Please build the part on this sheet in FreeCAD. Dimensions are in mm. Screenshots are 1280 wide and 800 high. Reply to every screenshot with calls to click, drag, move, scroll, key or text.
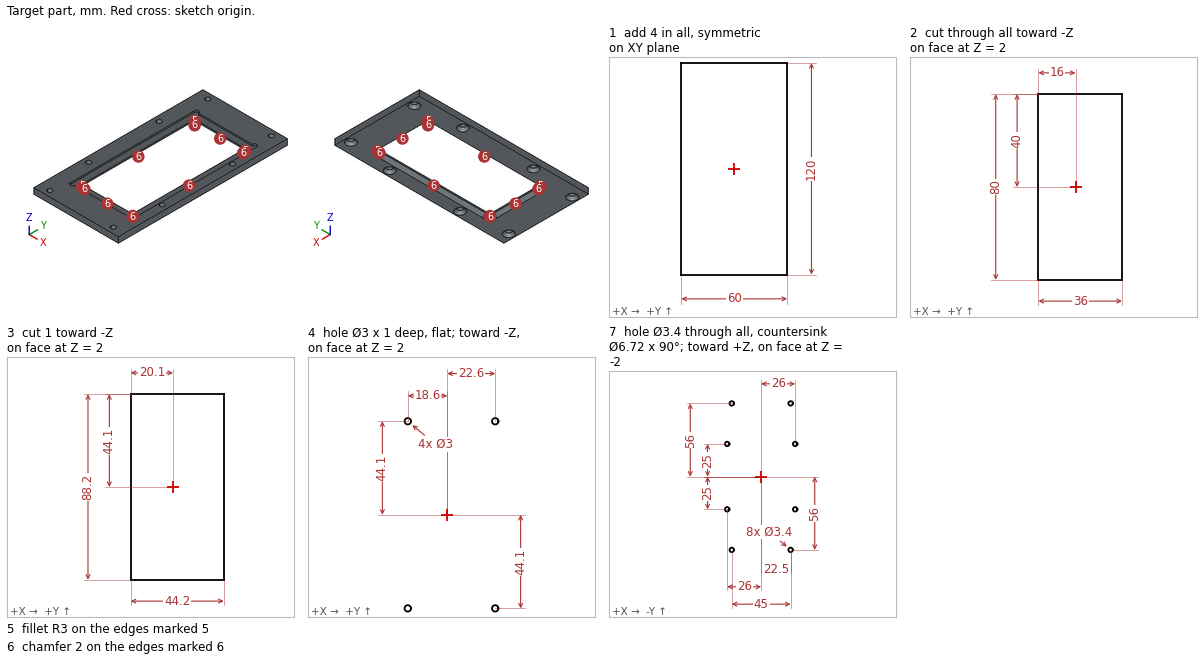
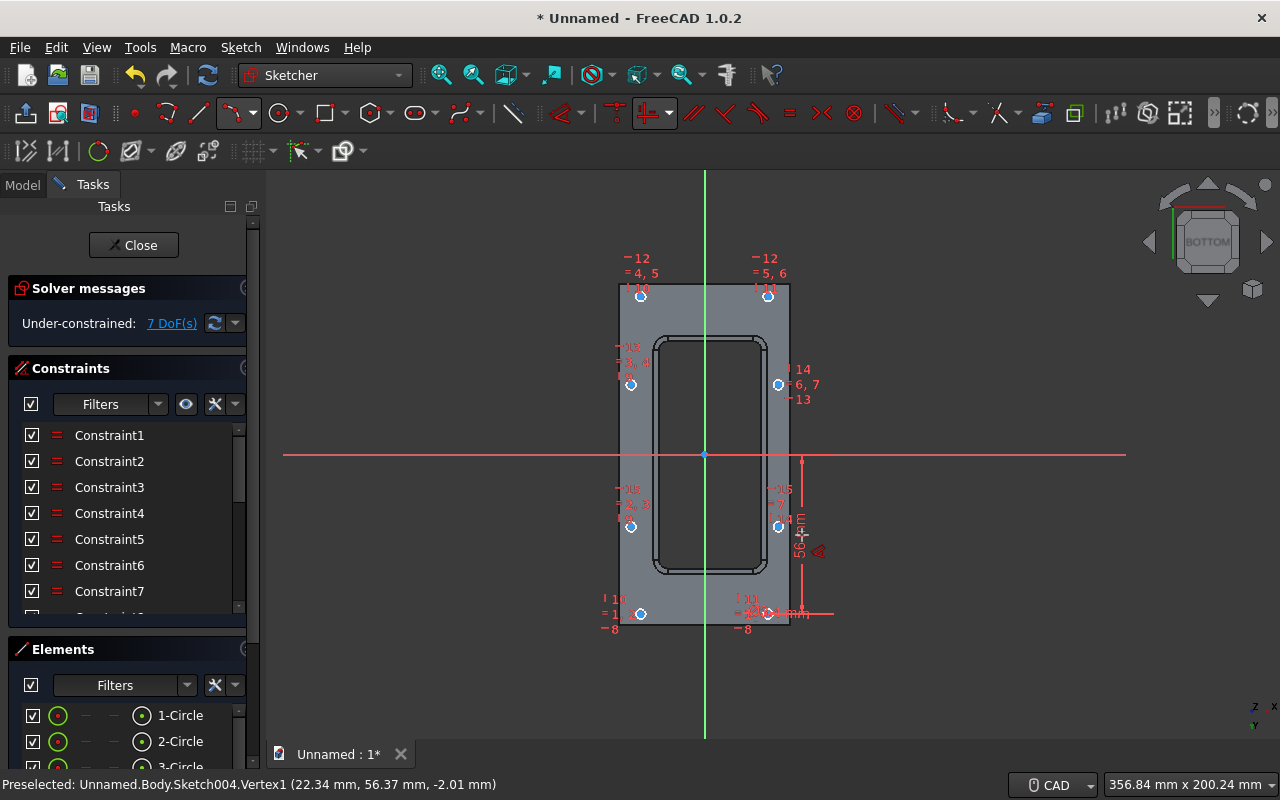
click(631, 527)
click(668, 561)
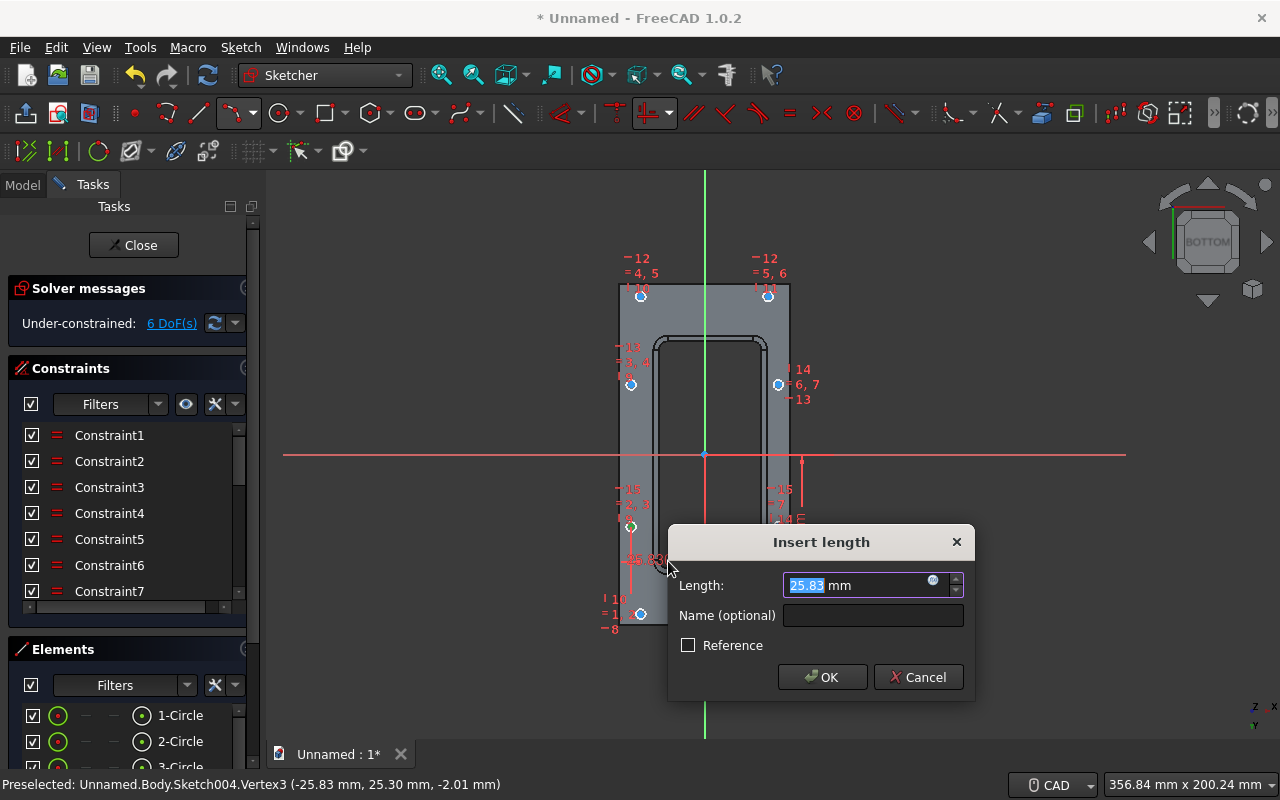
text(26)
key(Return)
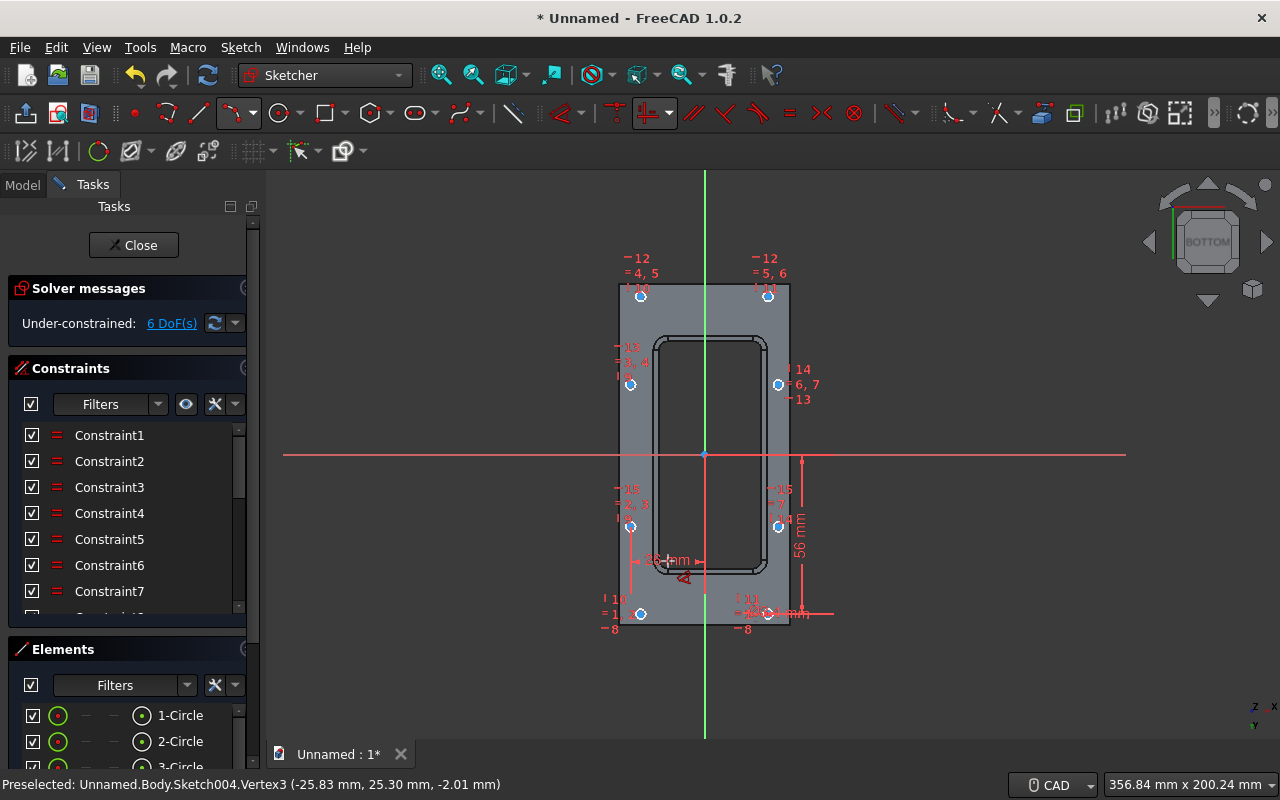
click(631, 527)
click(597, 491)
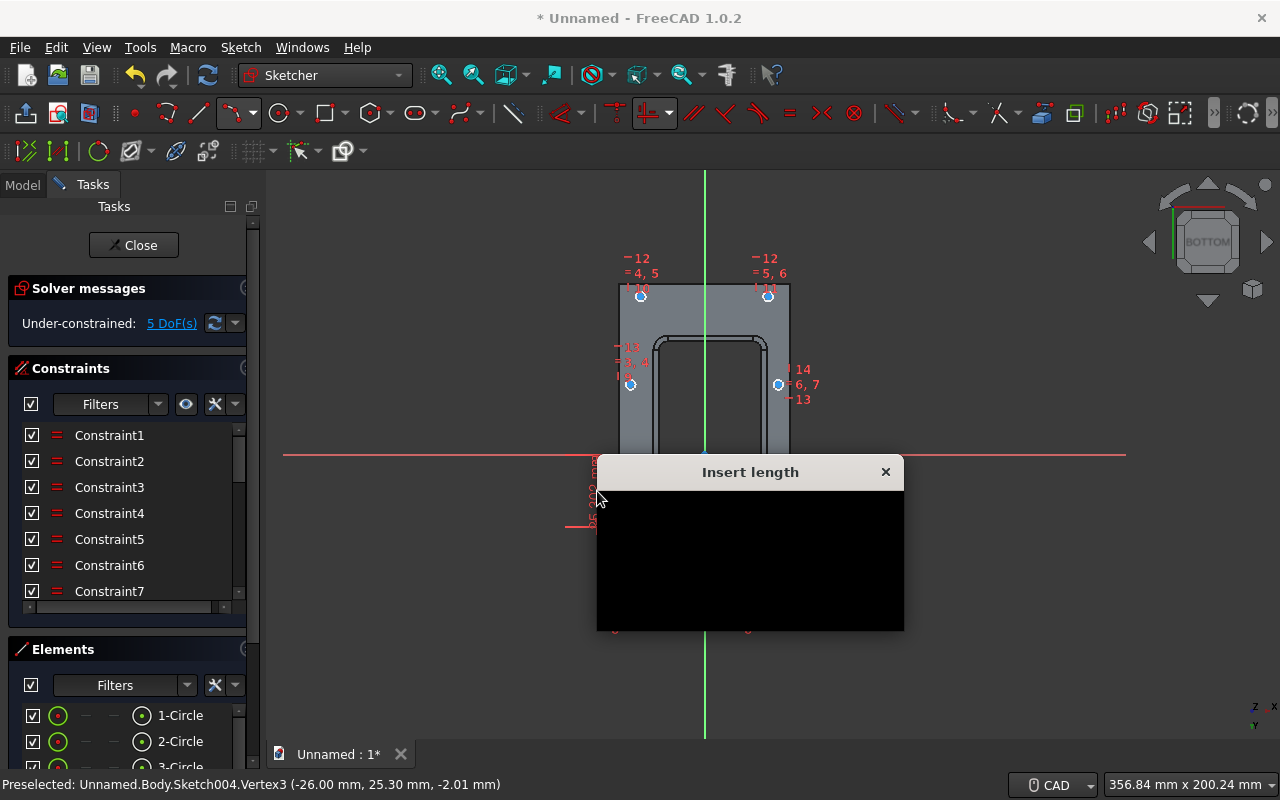
text(25)
key(Return)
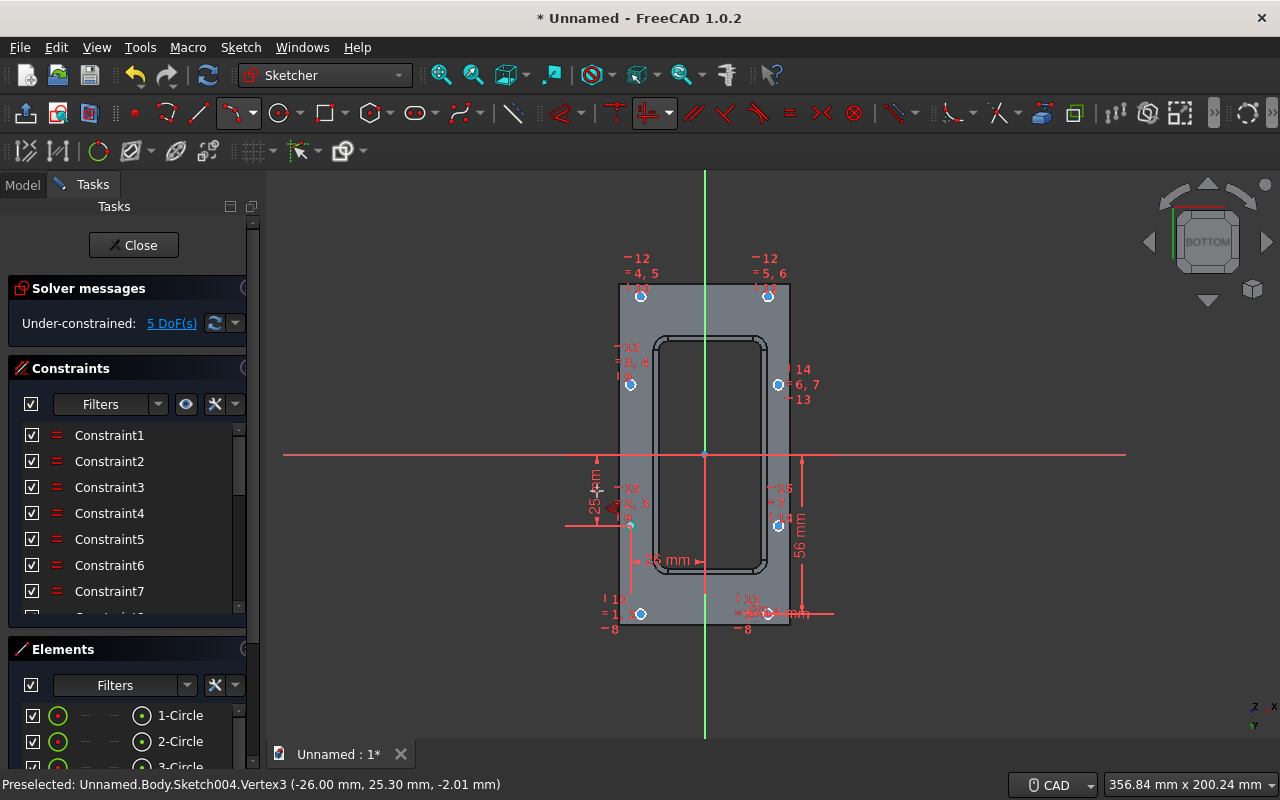
click(631, 385)
click(597, 420)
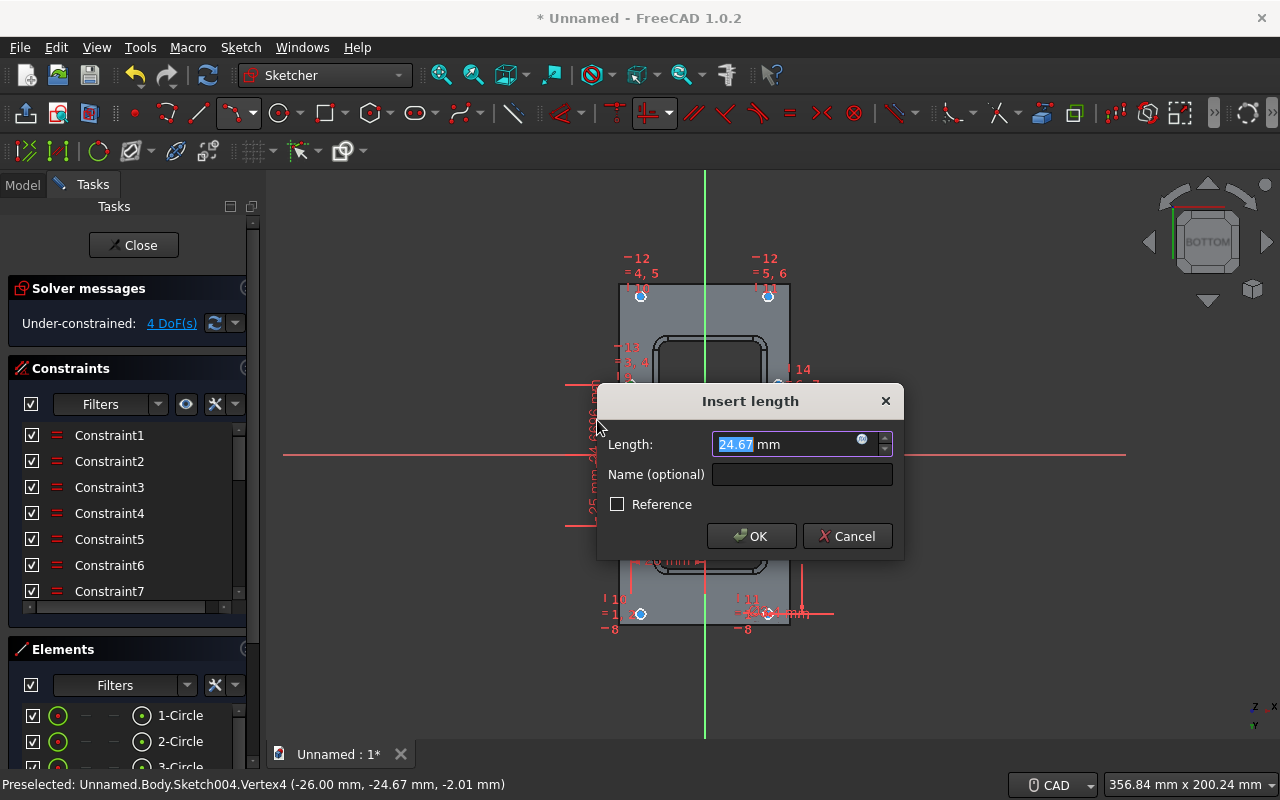
text(25)
key(Return)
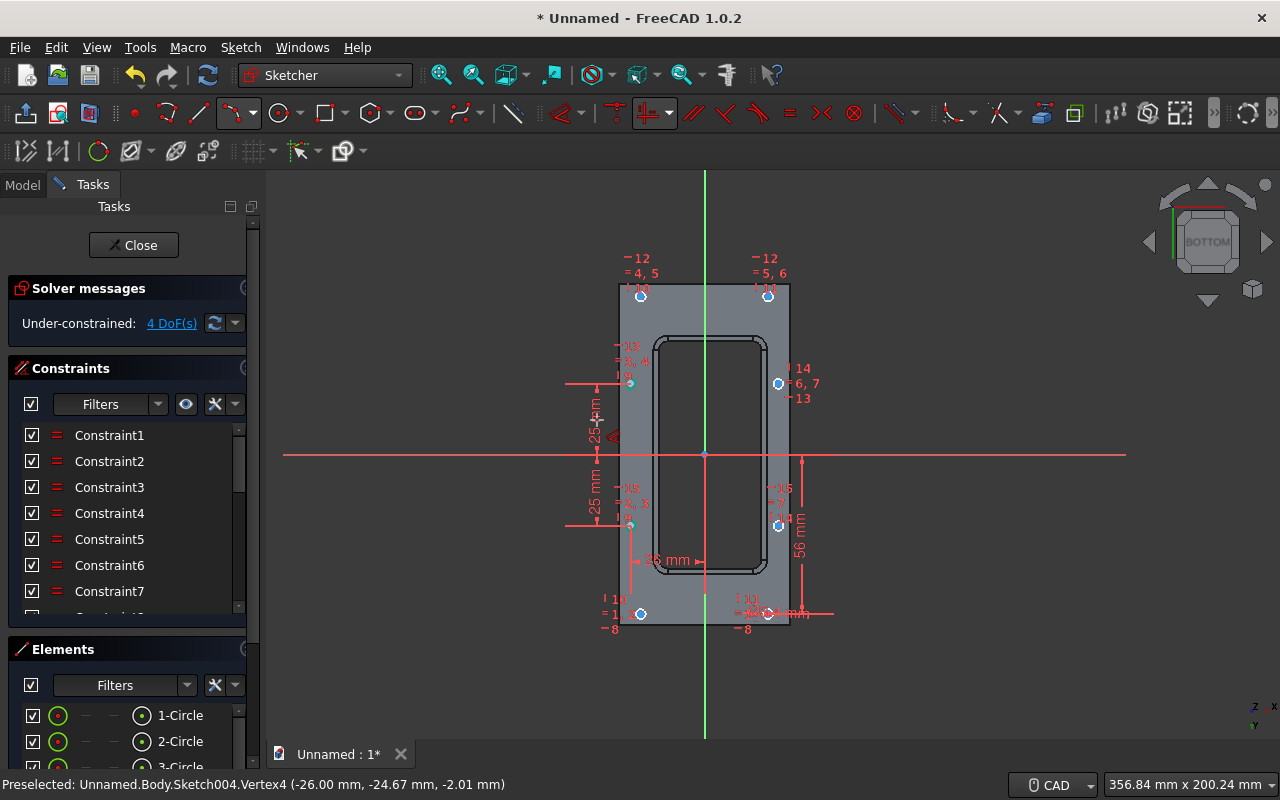
click(641, 297)
click(607, 376)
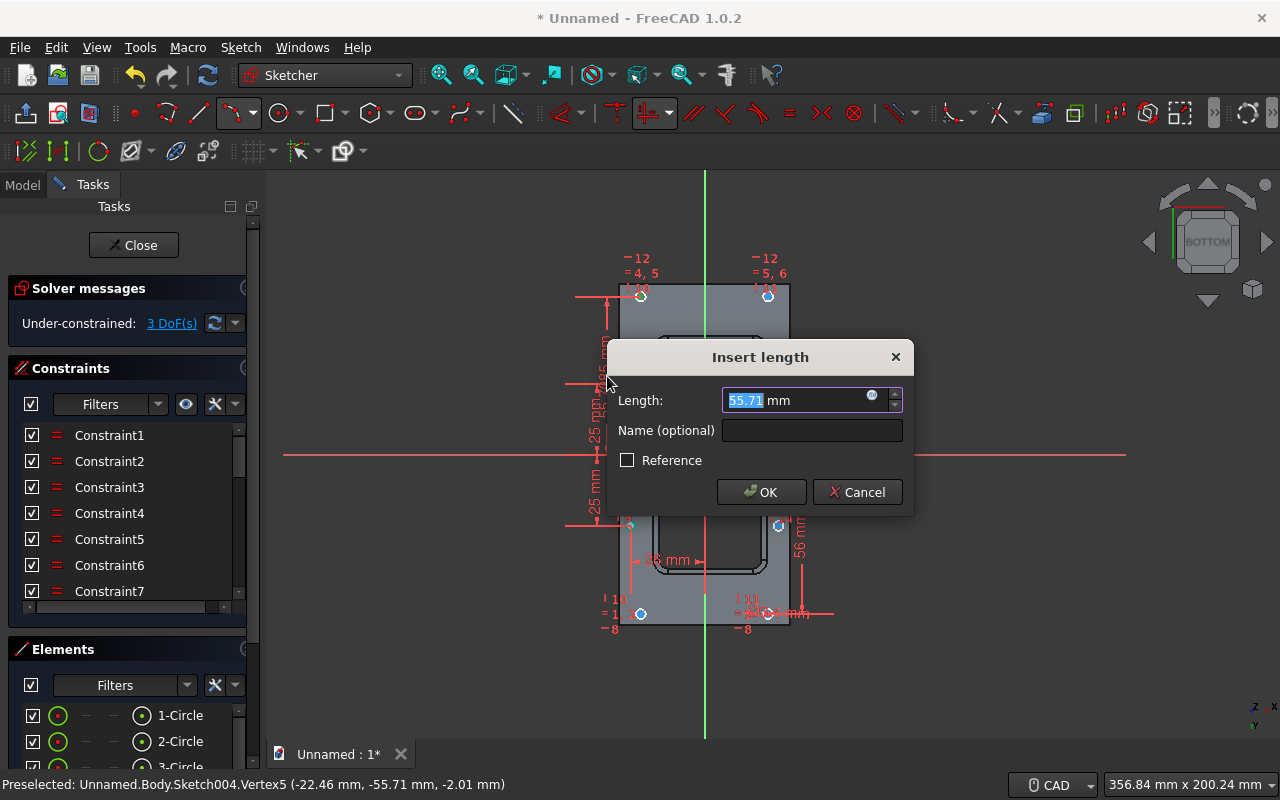
text(56)
key(Return)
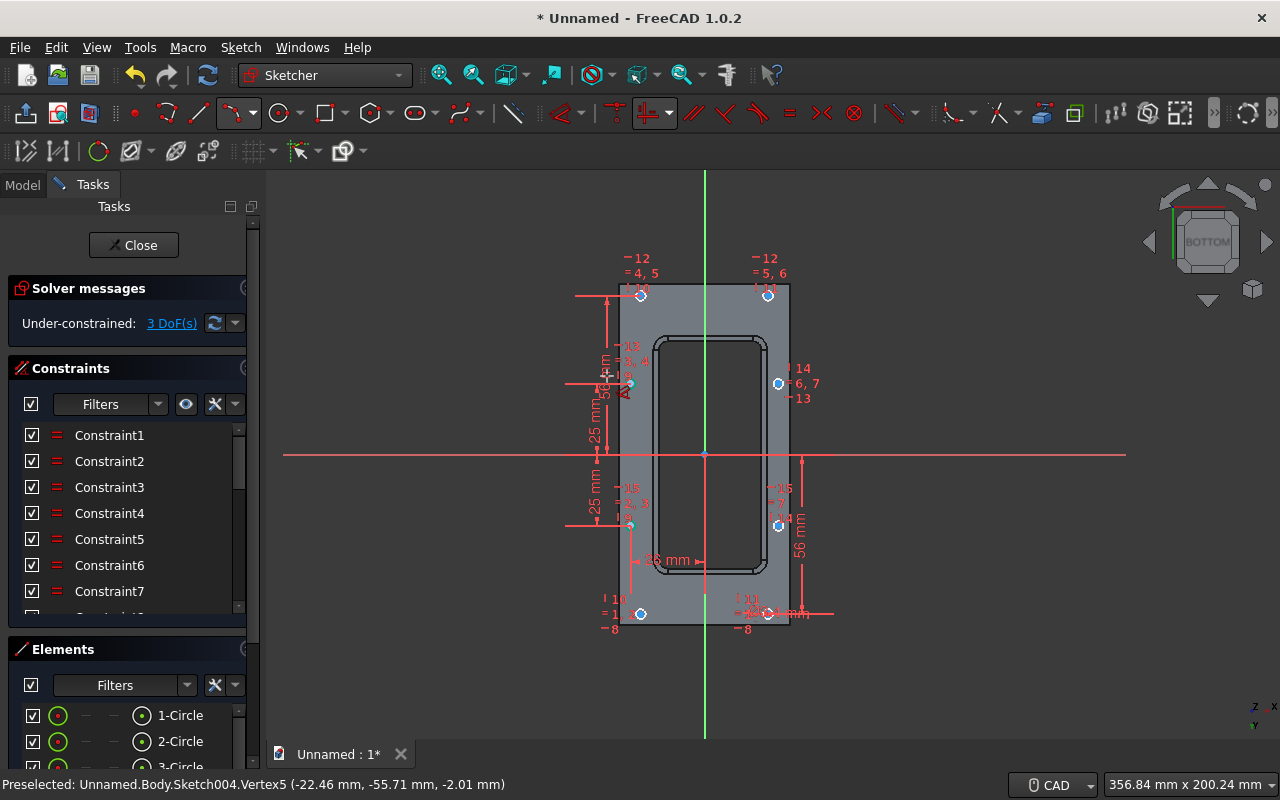
click(778, 384)
click(741, 350)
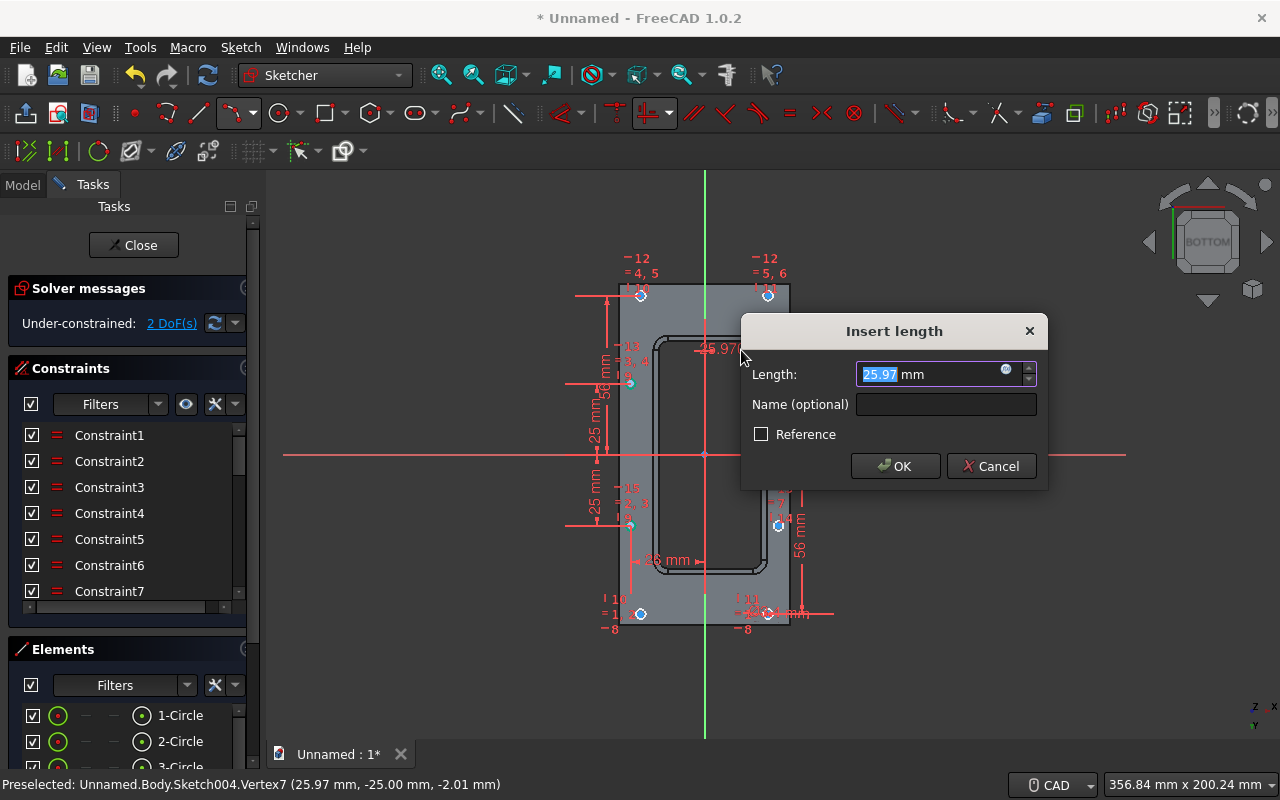
text(26)
key(Return)